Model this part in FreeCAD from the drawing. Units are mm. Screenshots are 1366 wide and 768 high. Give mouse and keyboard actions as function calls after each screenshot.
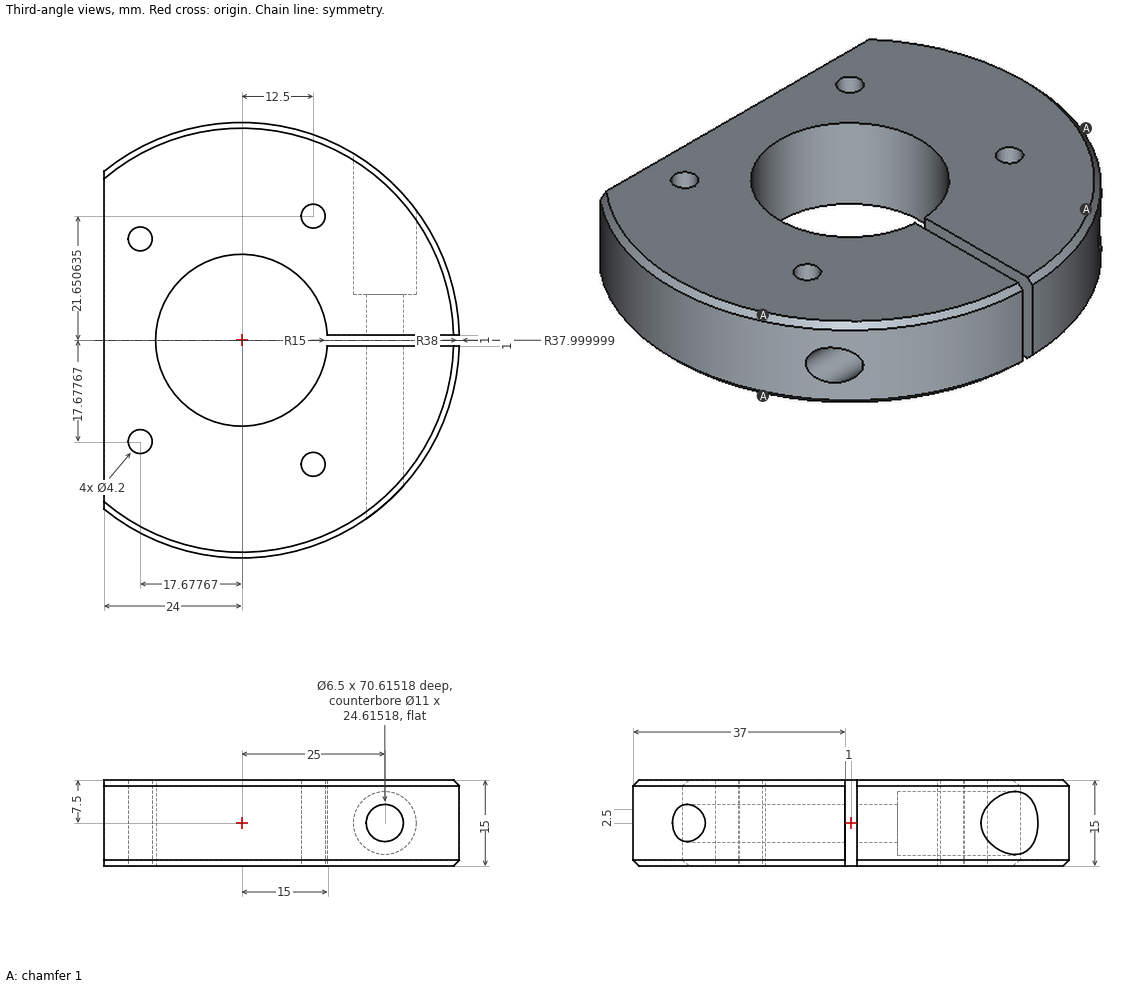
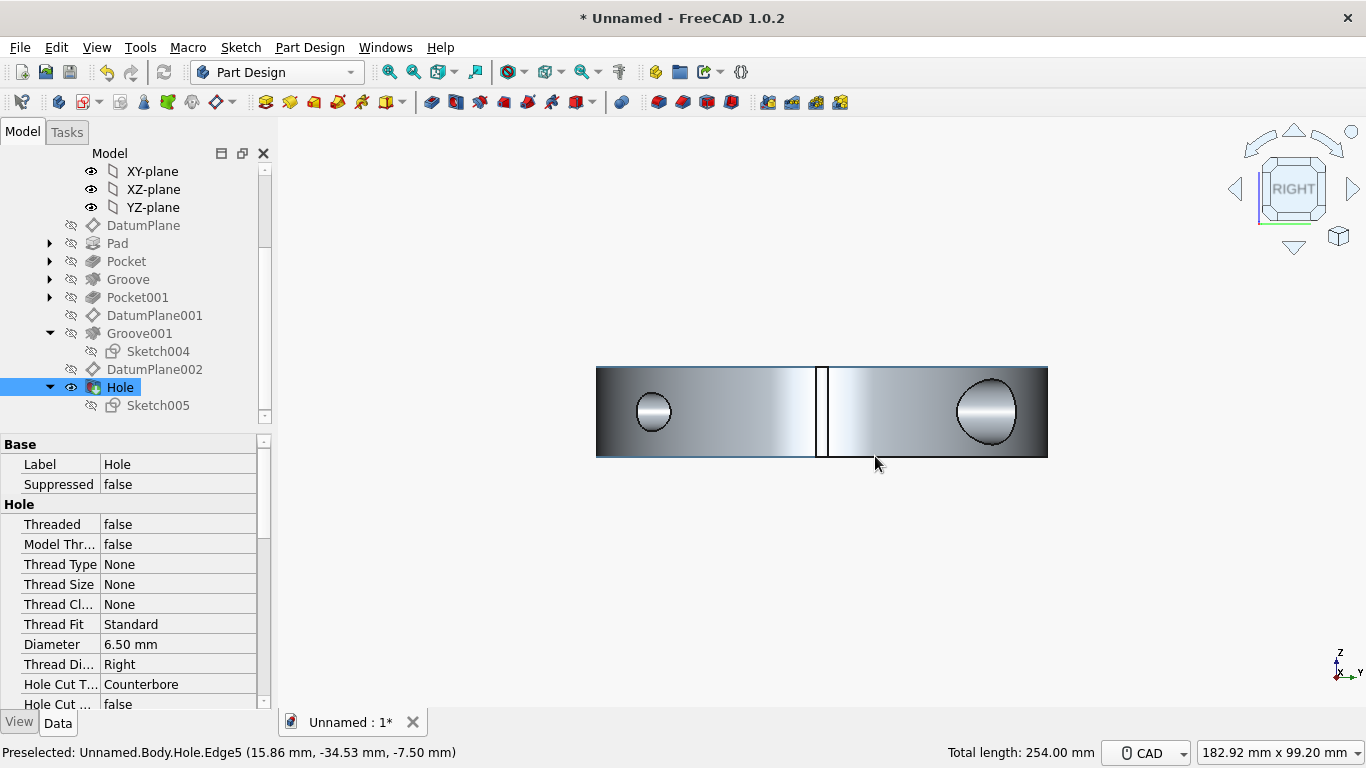
key(v)
key(f)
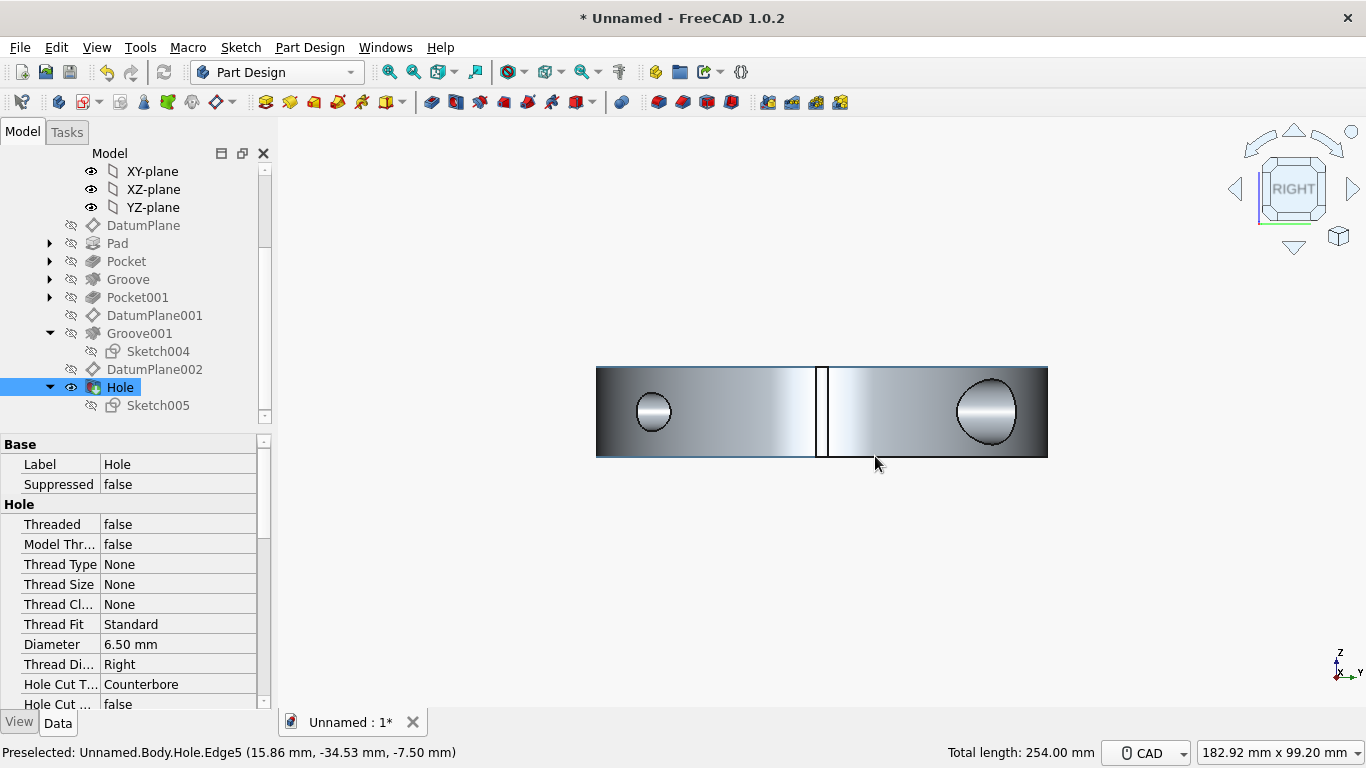
click(1027, 456, ctrl)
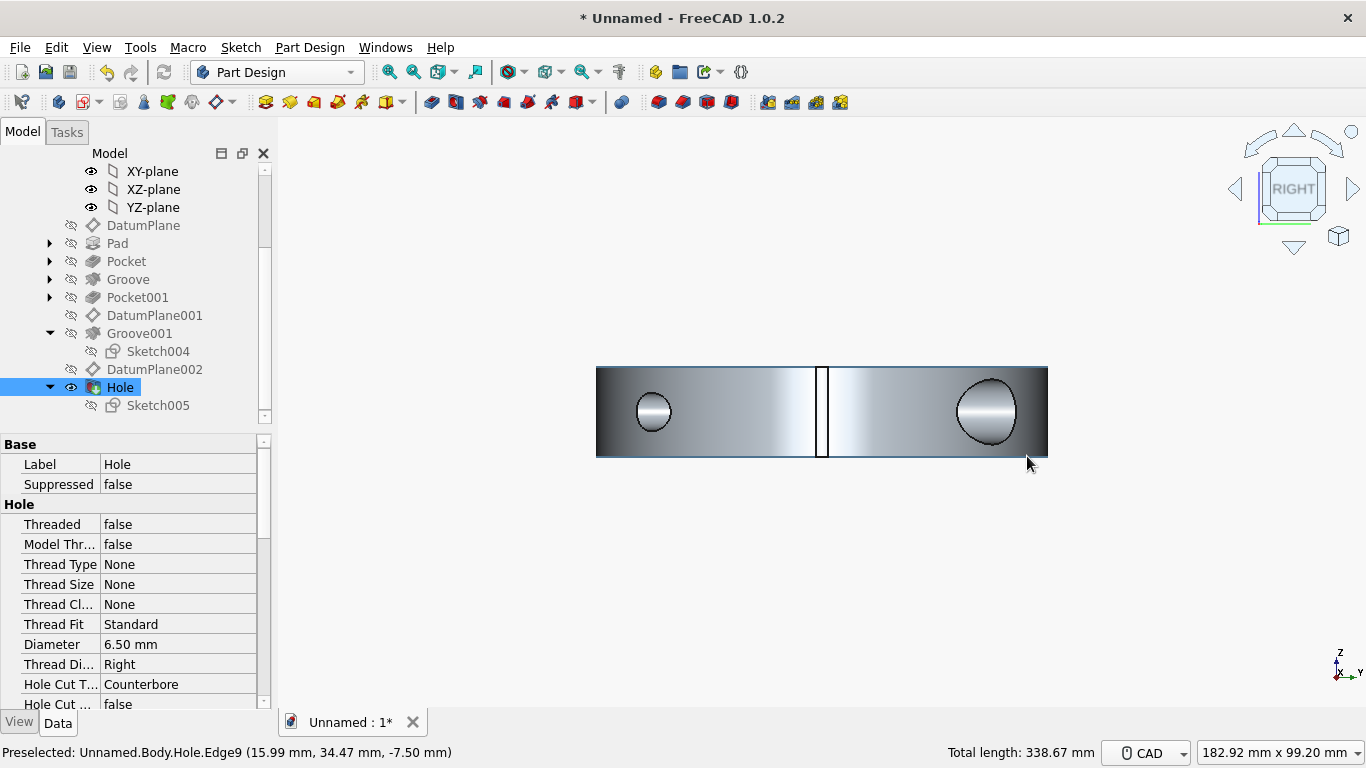
click(684, 102)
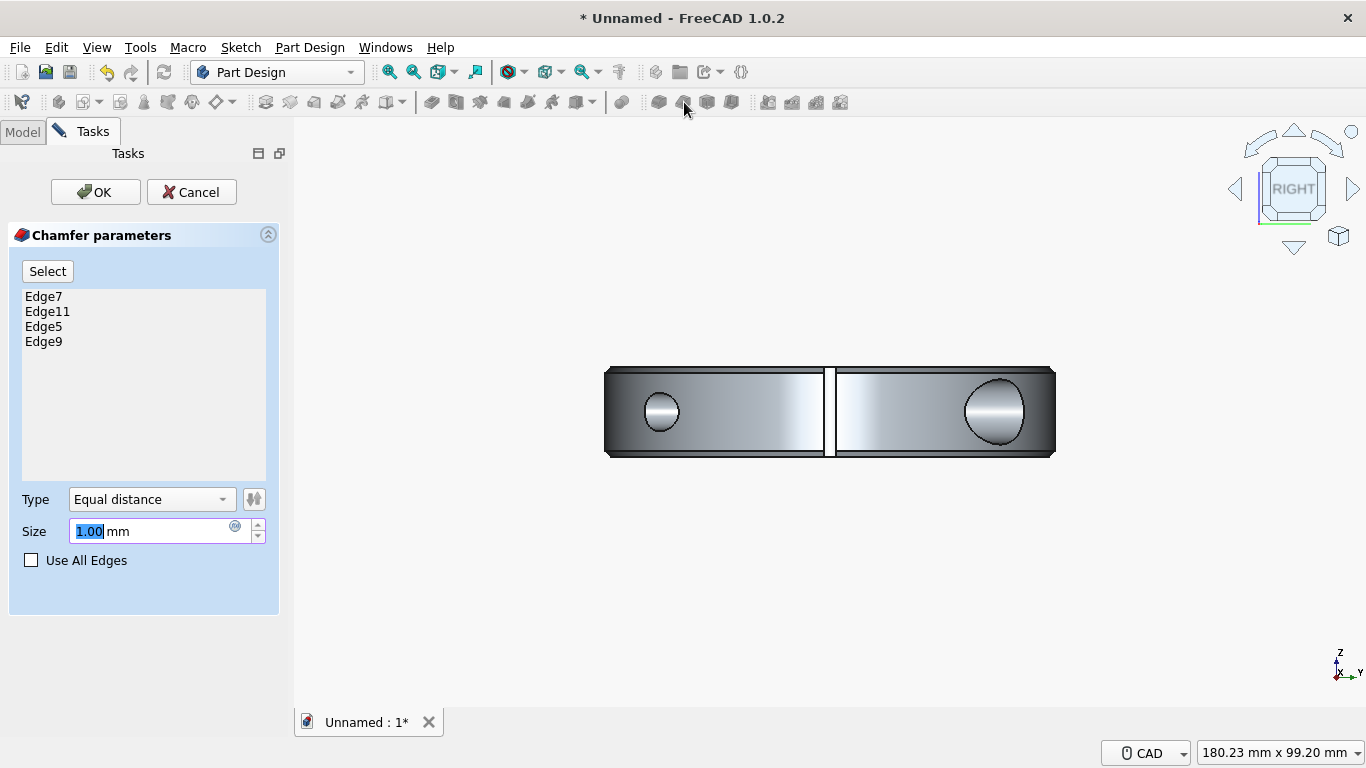
text(1)
key(Tab)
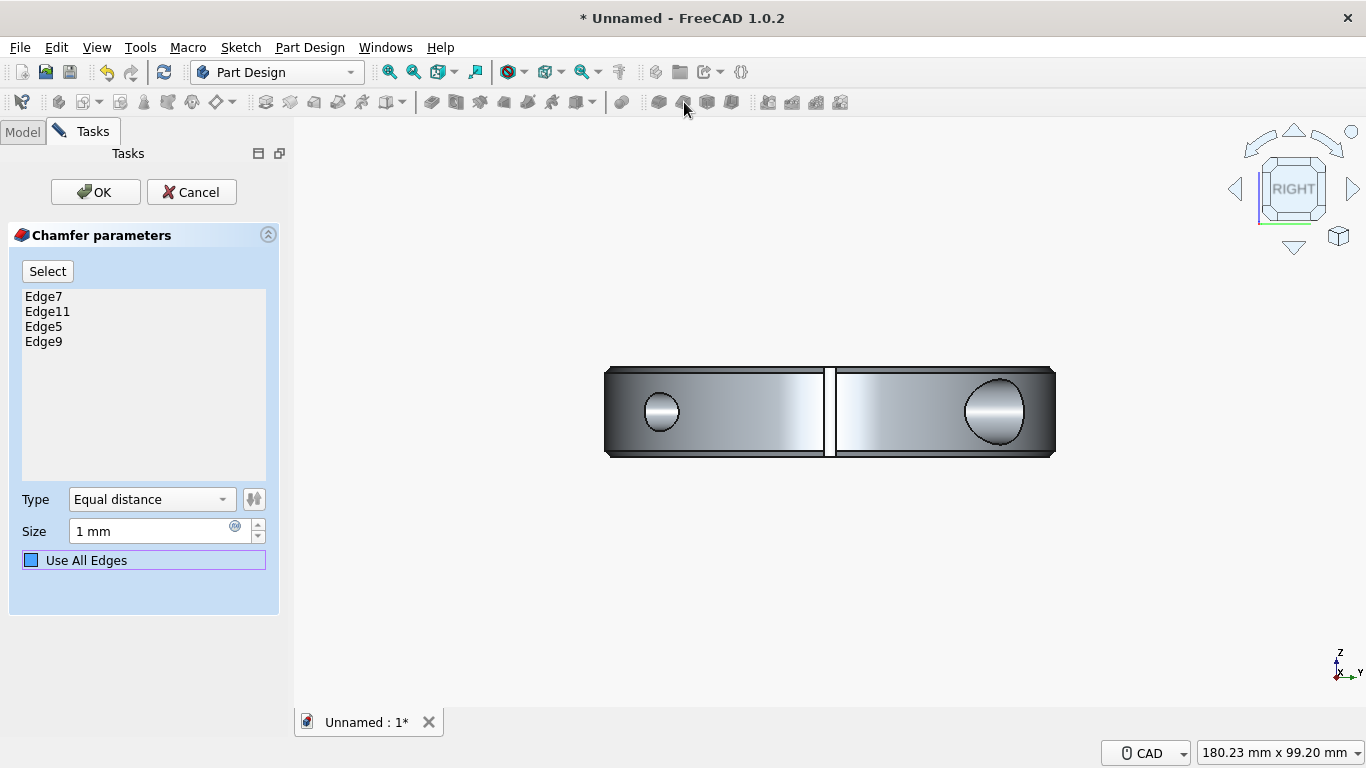
click(96, 192)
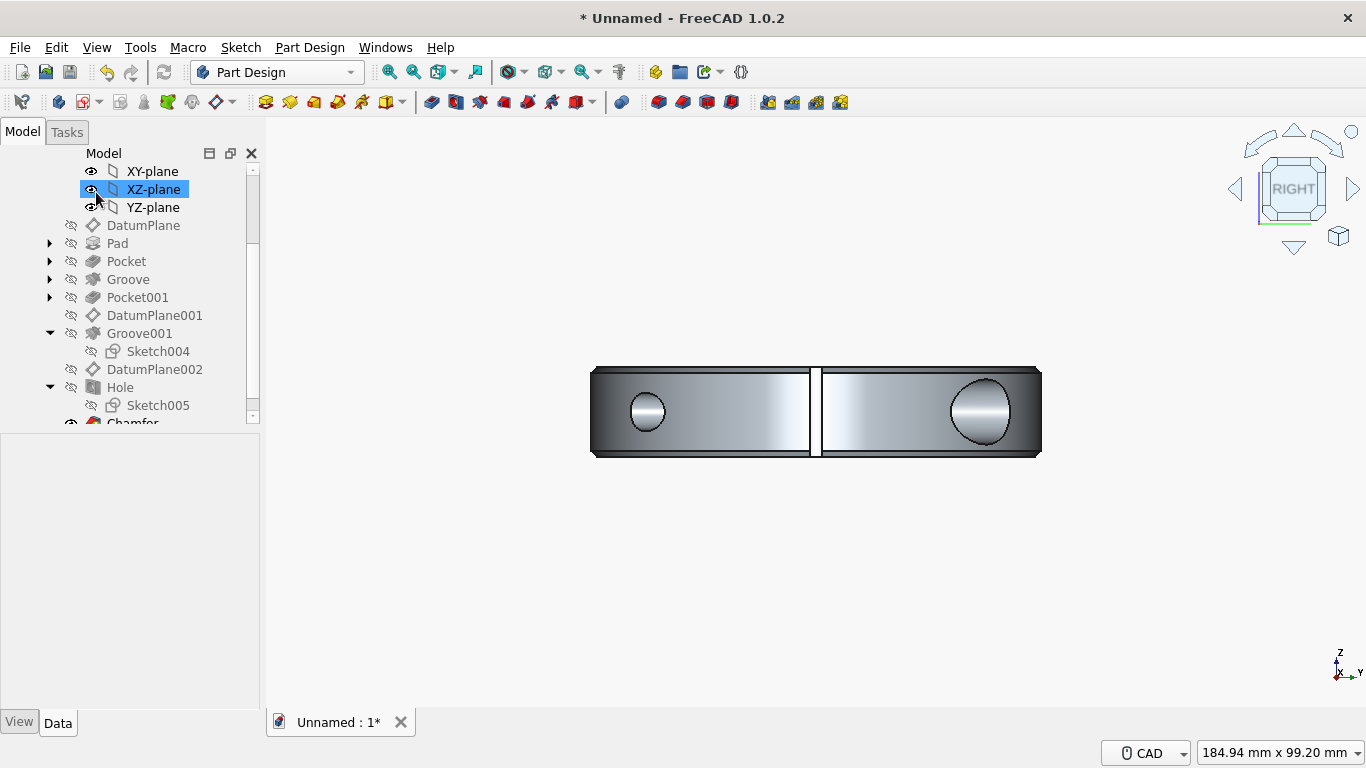
key(0)